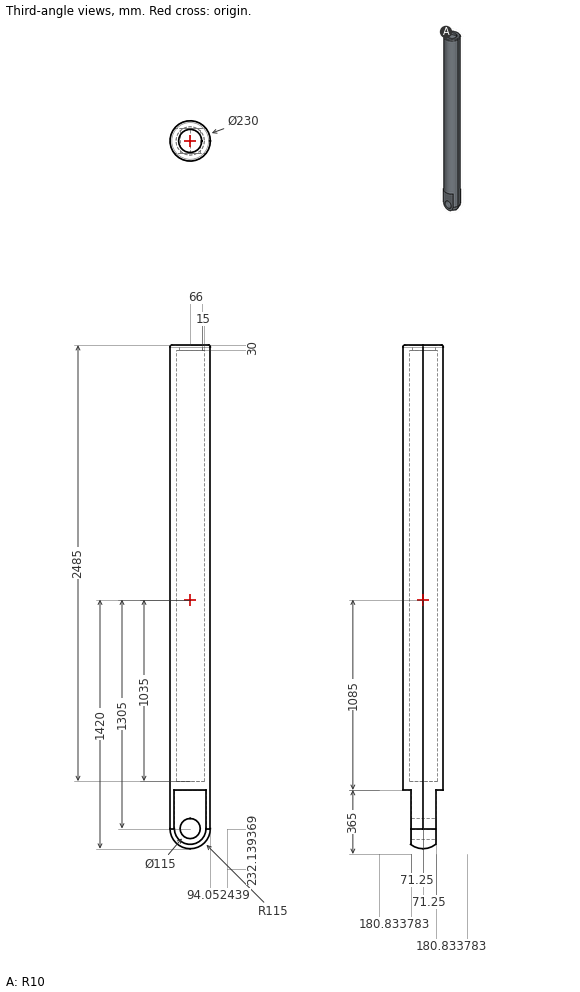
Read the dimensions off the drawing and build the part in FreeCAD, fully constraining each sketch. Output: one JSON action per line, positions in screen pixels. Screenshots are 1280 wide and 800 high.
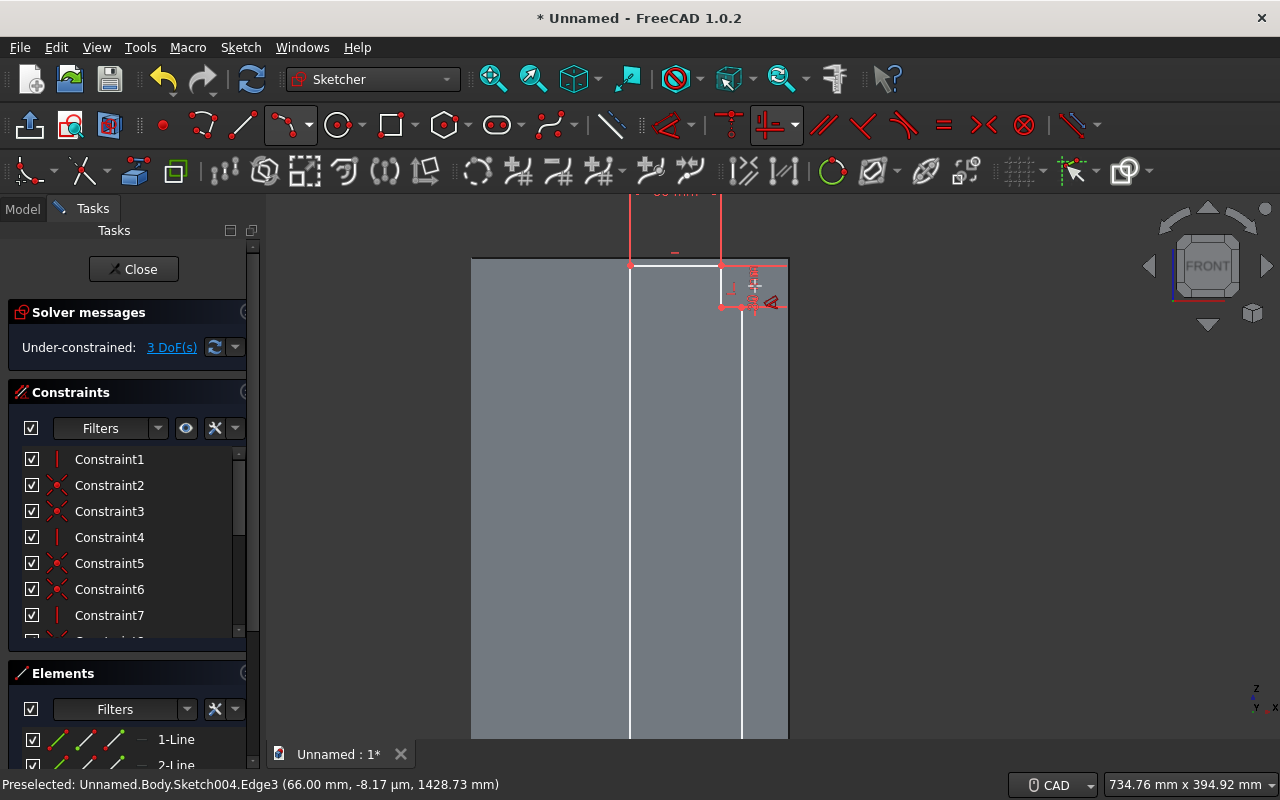
{"action": "scroll", "coordinate": [731, 307], "scroll_direction": "up", "scroll_amount": 4}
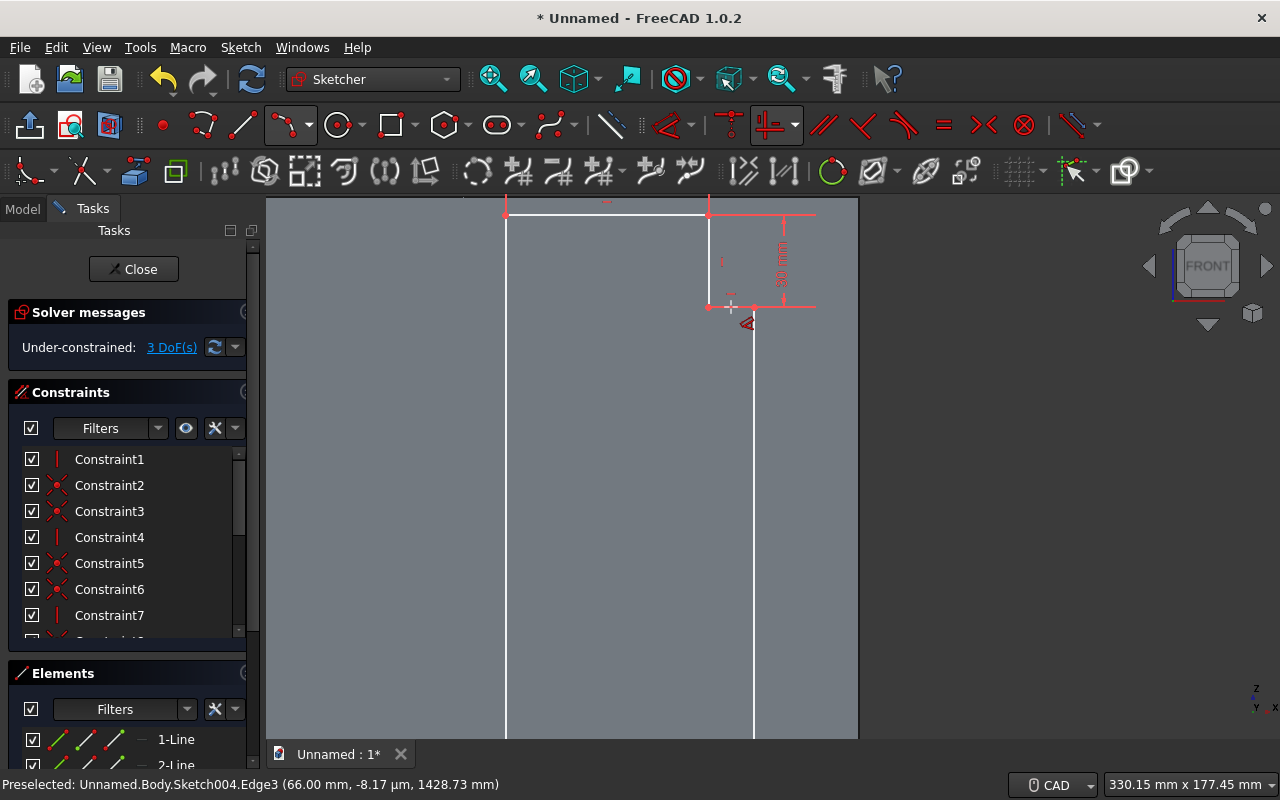
{"action": "left_click", "coordinate": [731, 307]}
{"action": "left_click", "coordinate": [731, 341]}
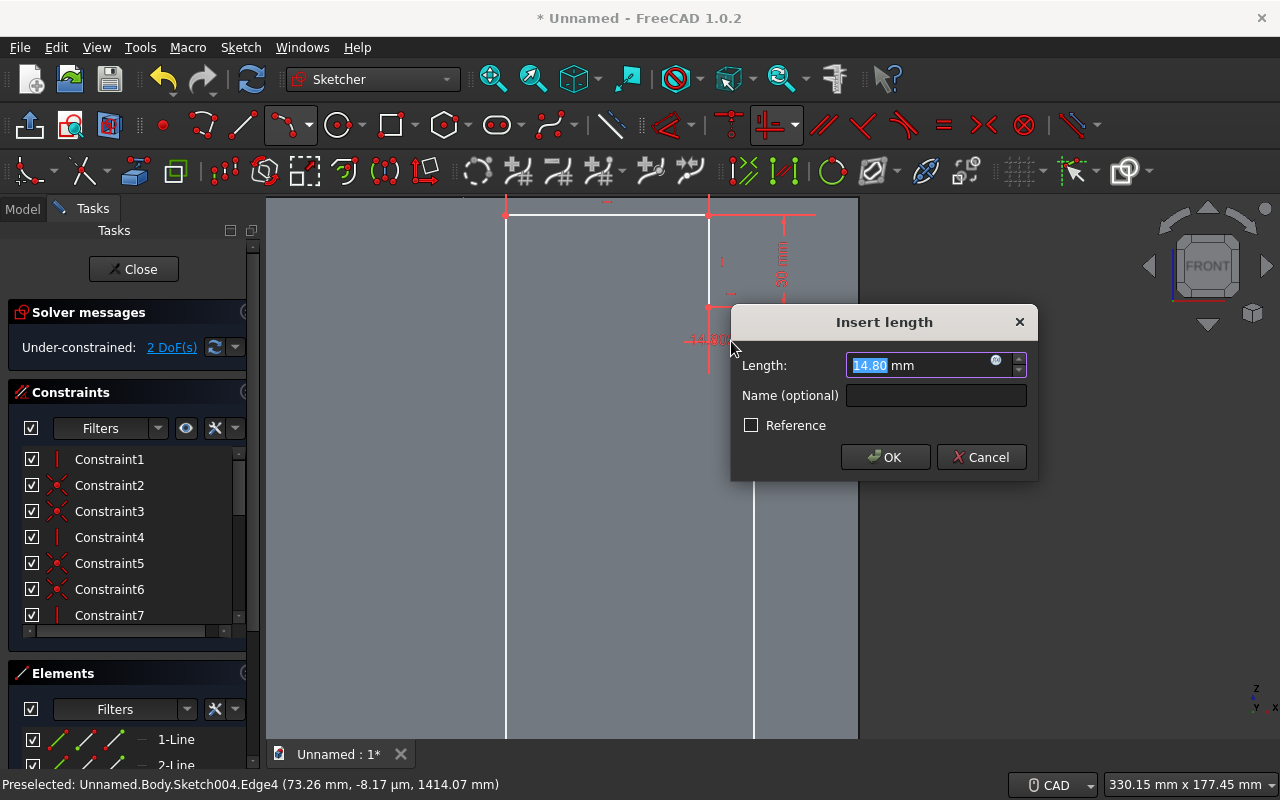
{"action": "type", "text": "15"}
{"action": "key", "text": "Return"}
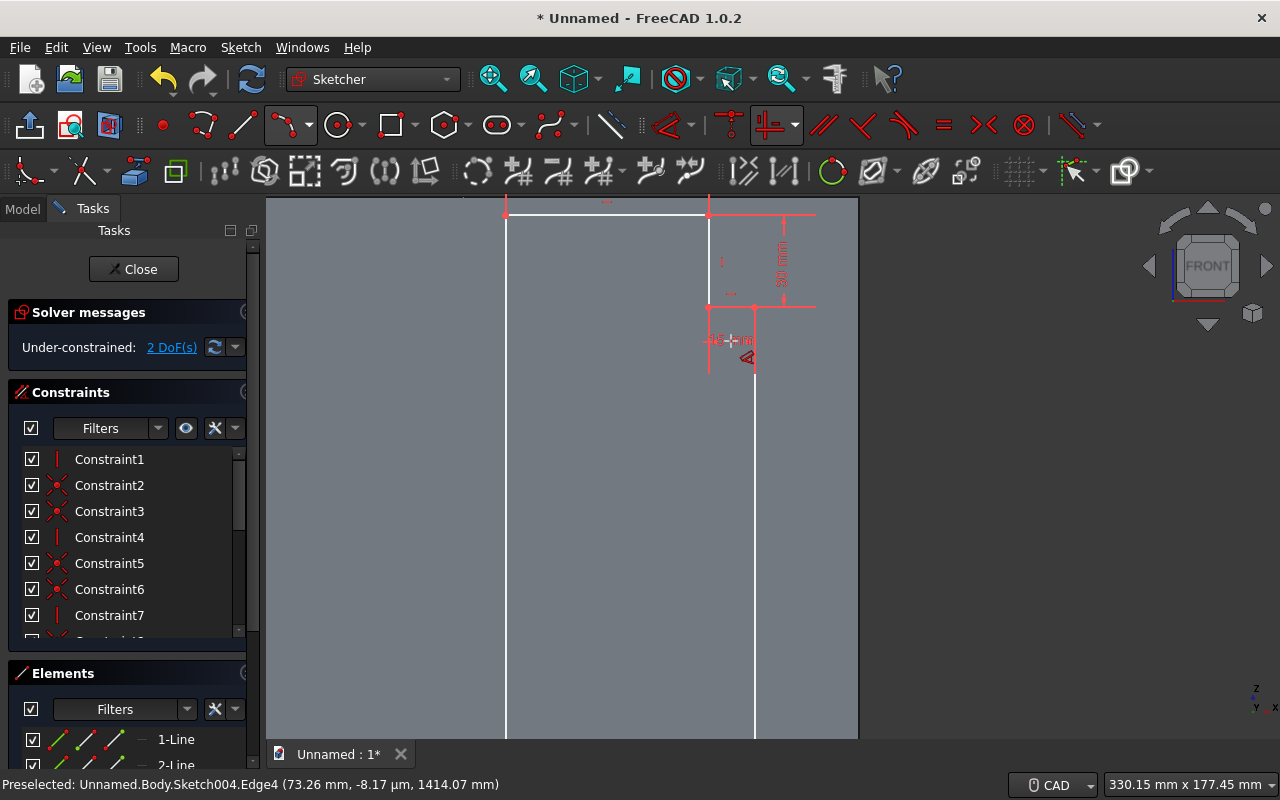
{"action": "scroll", "coordinate": [708, 281], "scroll_direction": "down", "scroll_amount": 15}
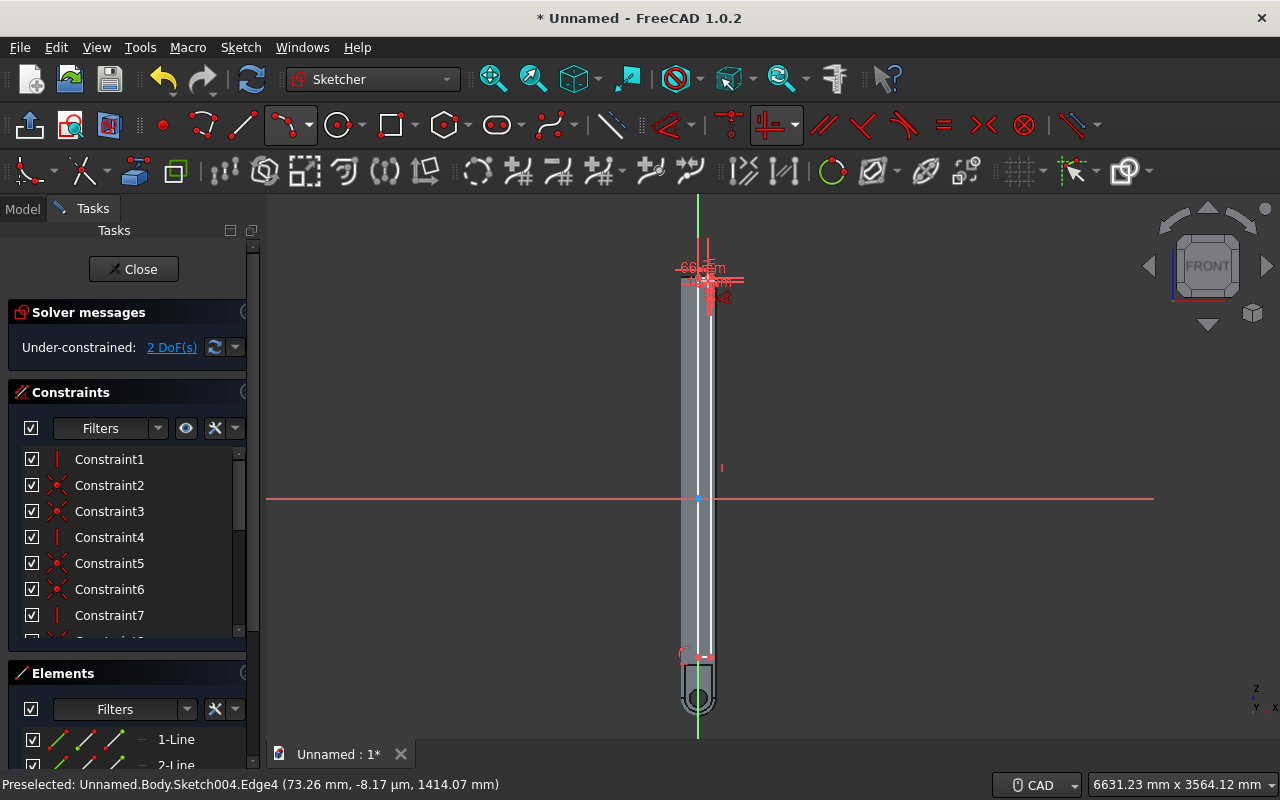
{"action": "left_click", "coordinate": [698, 543]}
{"action": "left_click", "coordinate": [664, 468]}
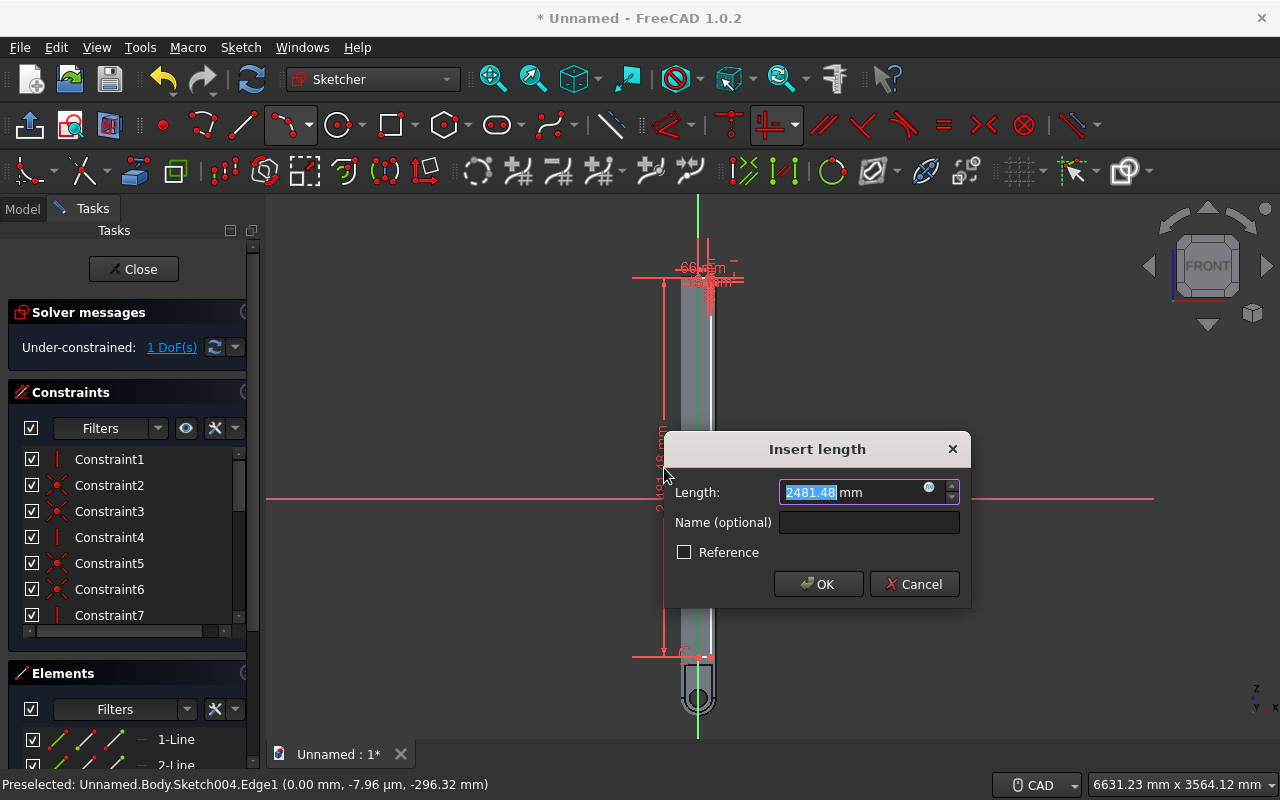
{"action": "type", "text": "2485"}
{"action": "key", "text": "Return"}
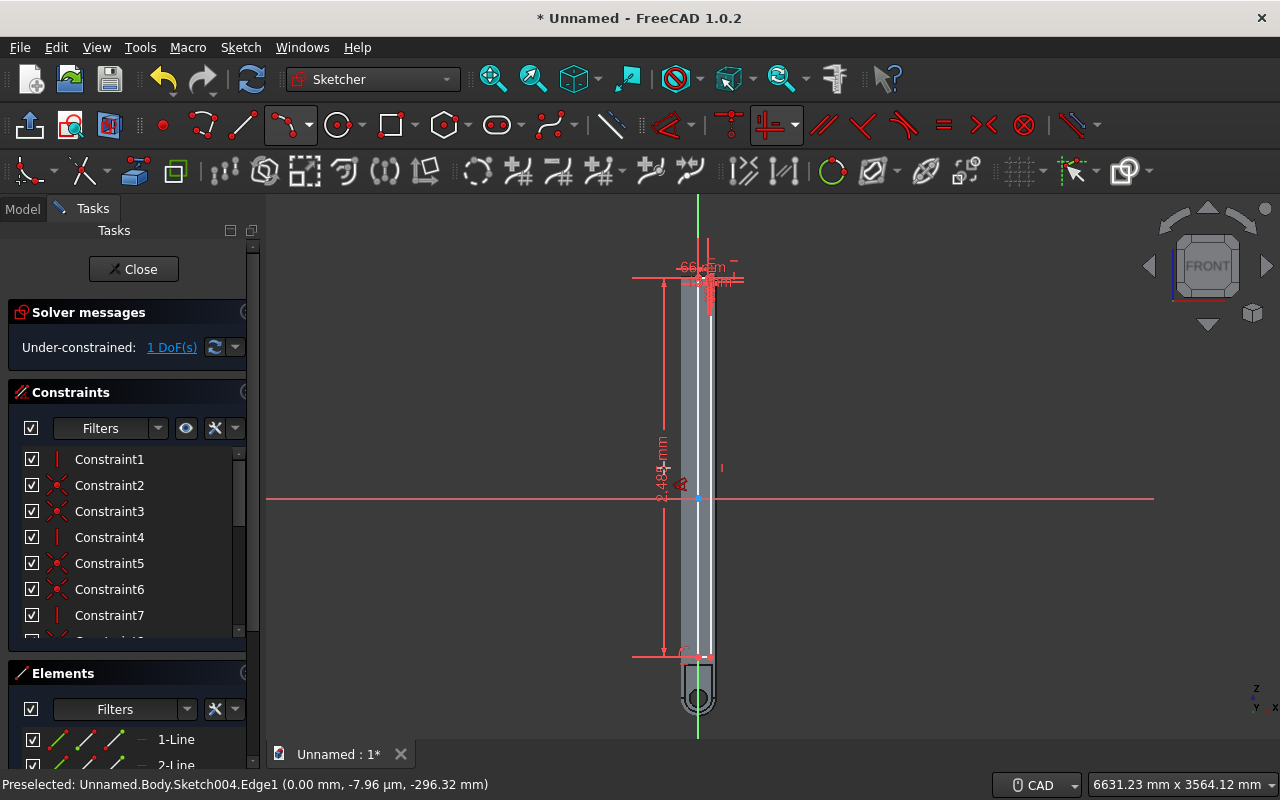
{"action": "left_click", "coordinate": [698, 657]}
{"action": "left_click", "coordinate": [664, 578]}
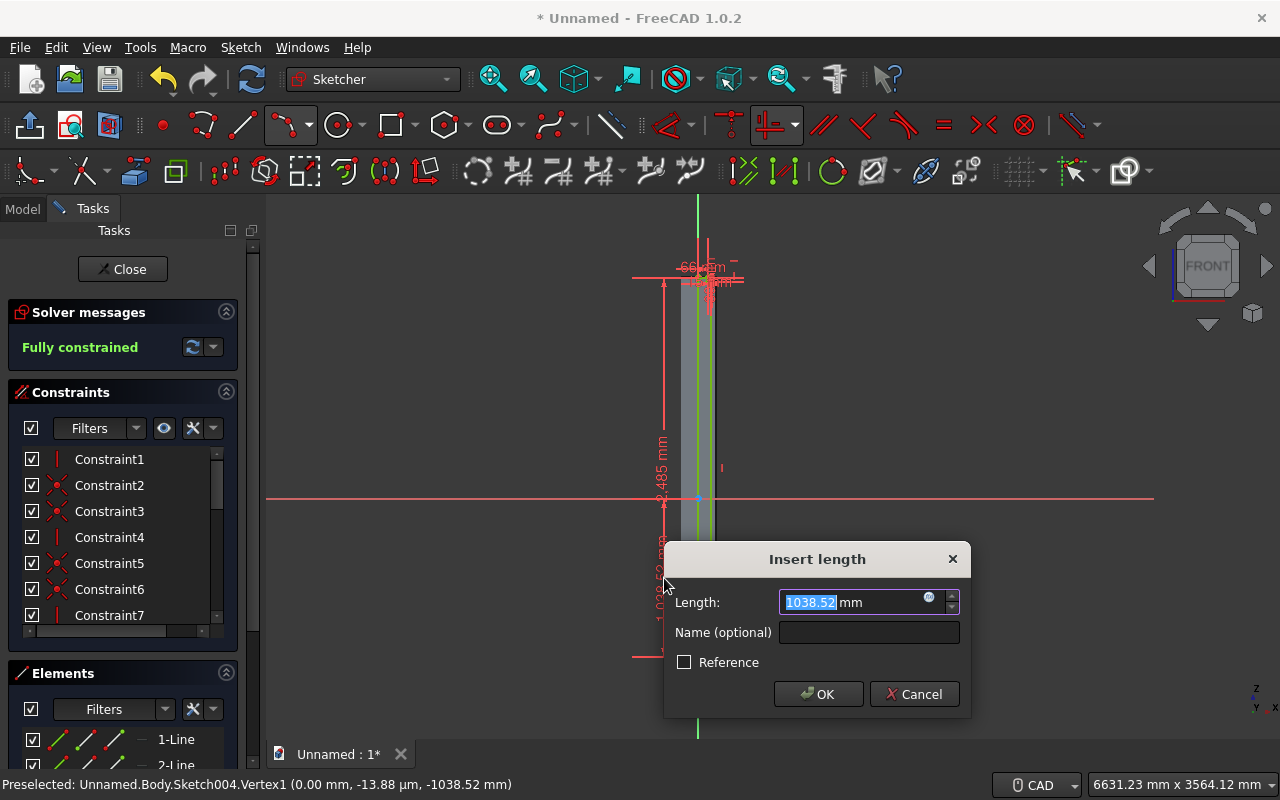
{"action": "type", "text": "1035"}
{"action": "key", "text": "Return"}
{"action": "key", "text": "Escape"}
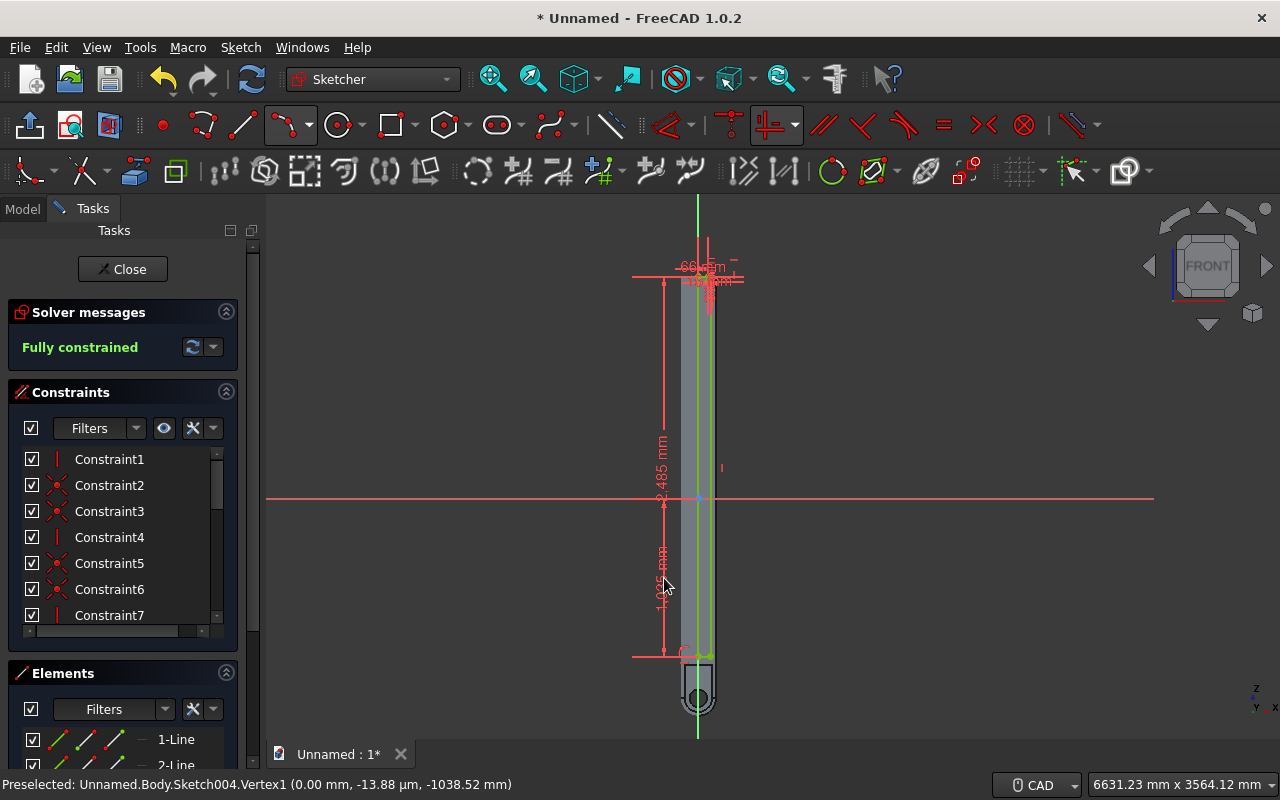
{"action": "left_click", "coordinate": [123, 269]}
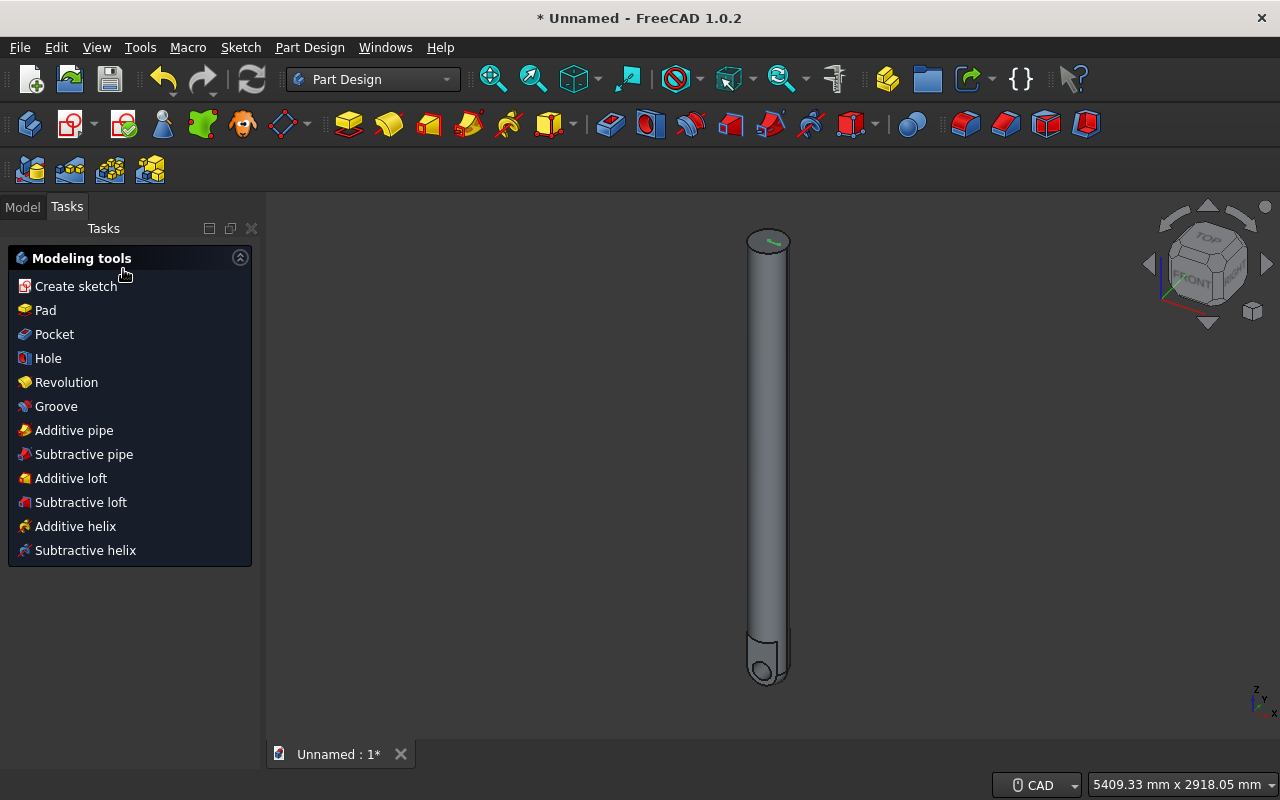
{"action": "left_click", "coordinate": [692, 124]}